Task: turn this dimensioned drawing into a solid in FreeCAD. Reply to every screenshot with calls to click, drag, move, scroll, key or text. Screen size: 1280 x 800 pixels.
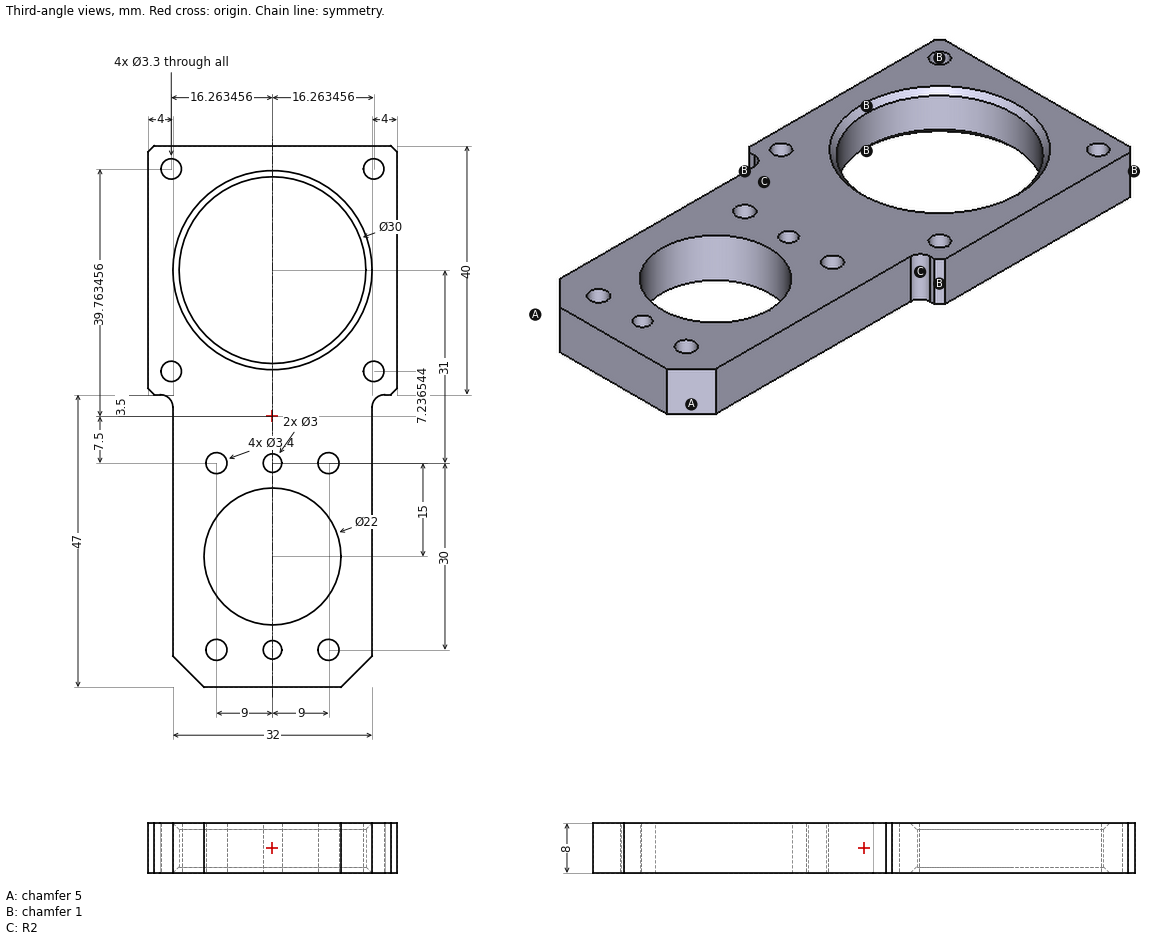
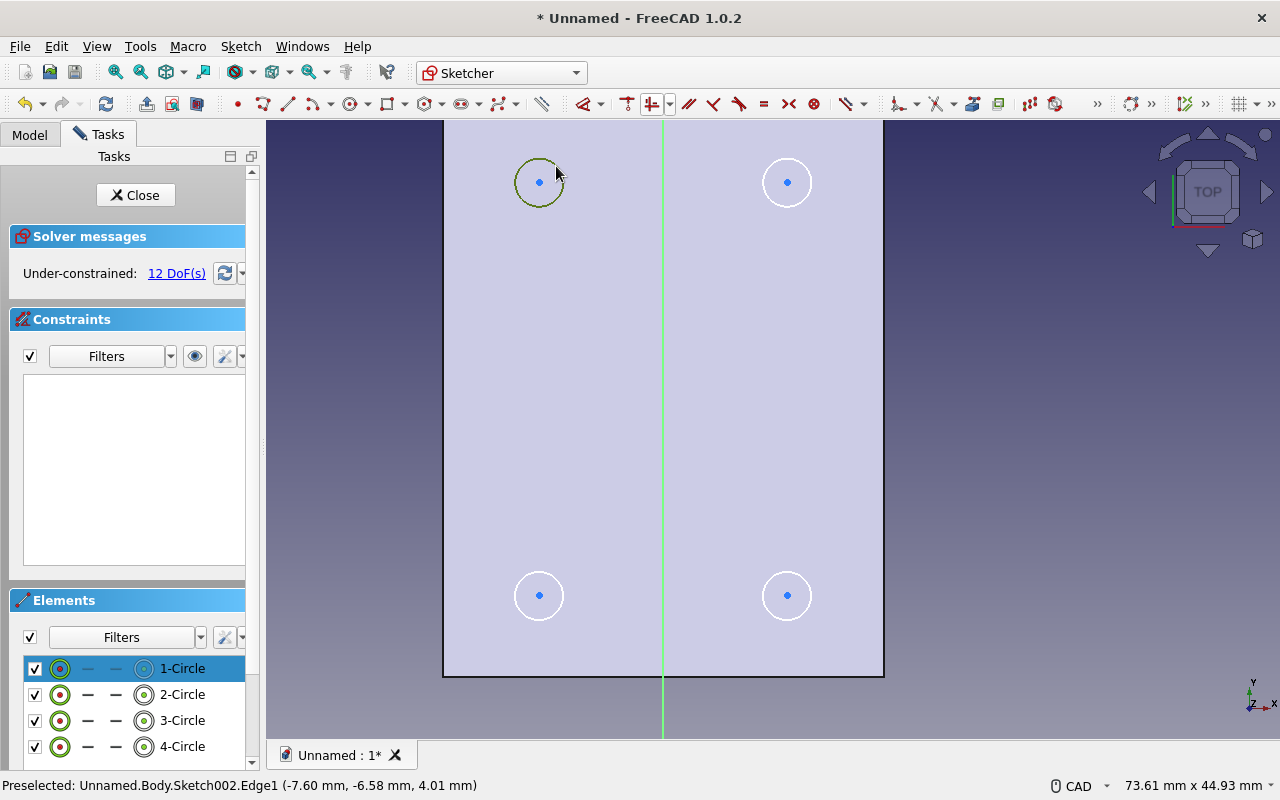
click(804, 166)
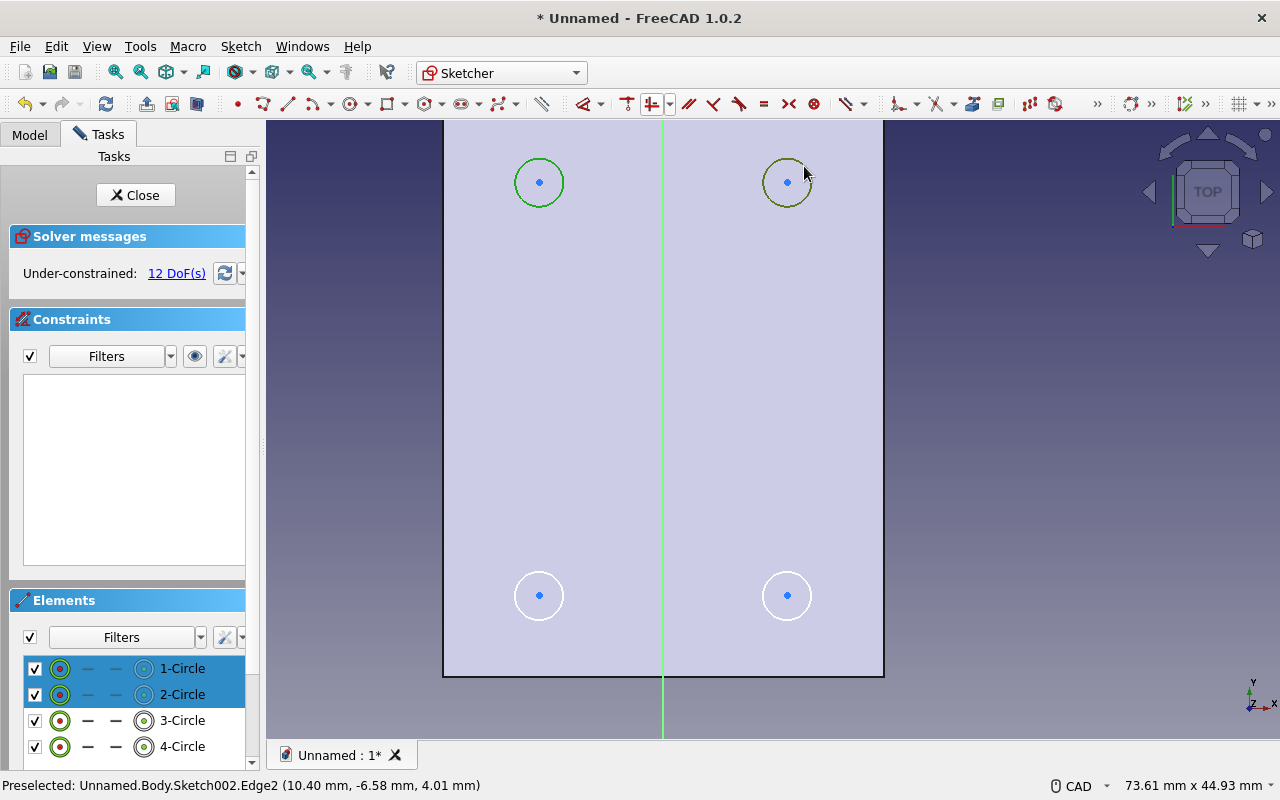
click(804, 579)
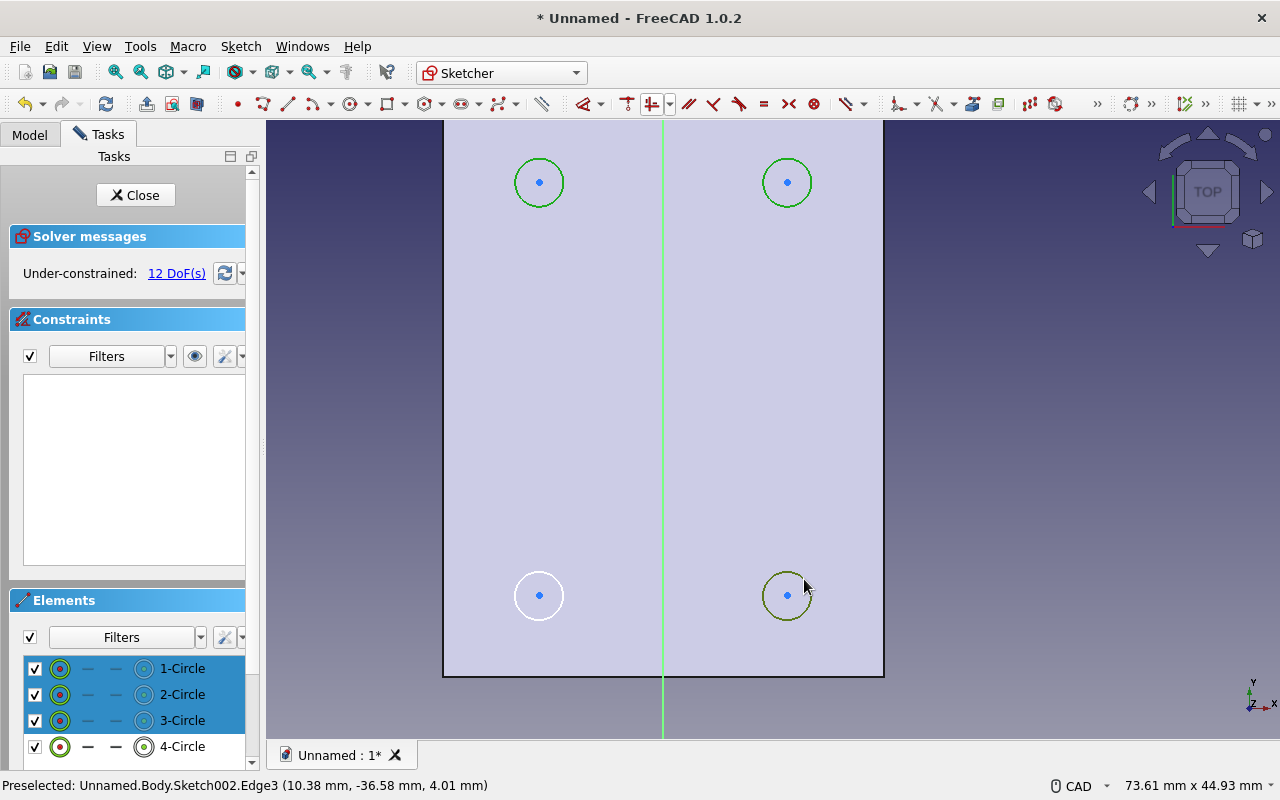
click(556, 579)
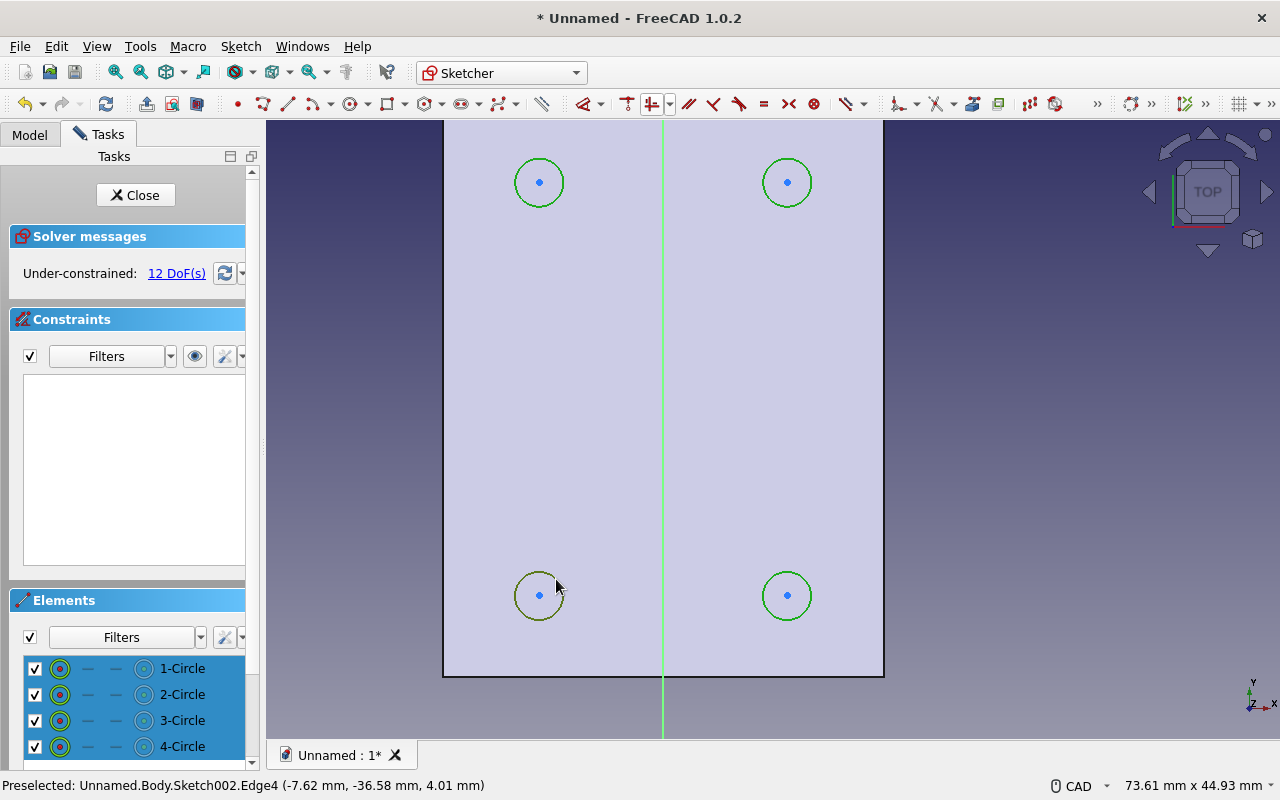
click(764, 104)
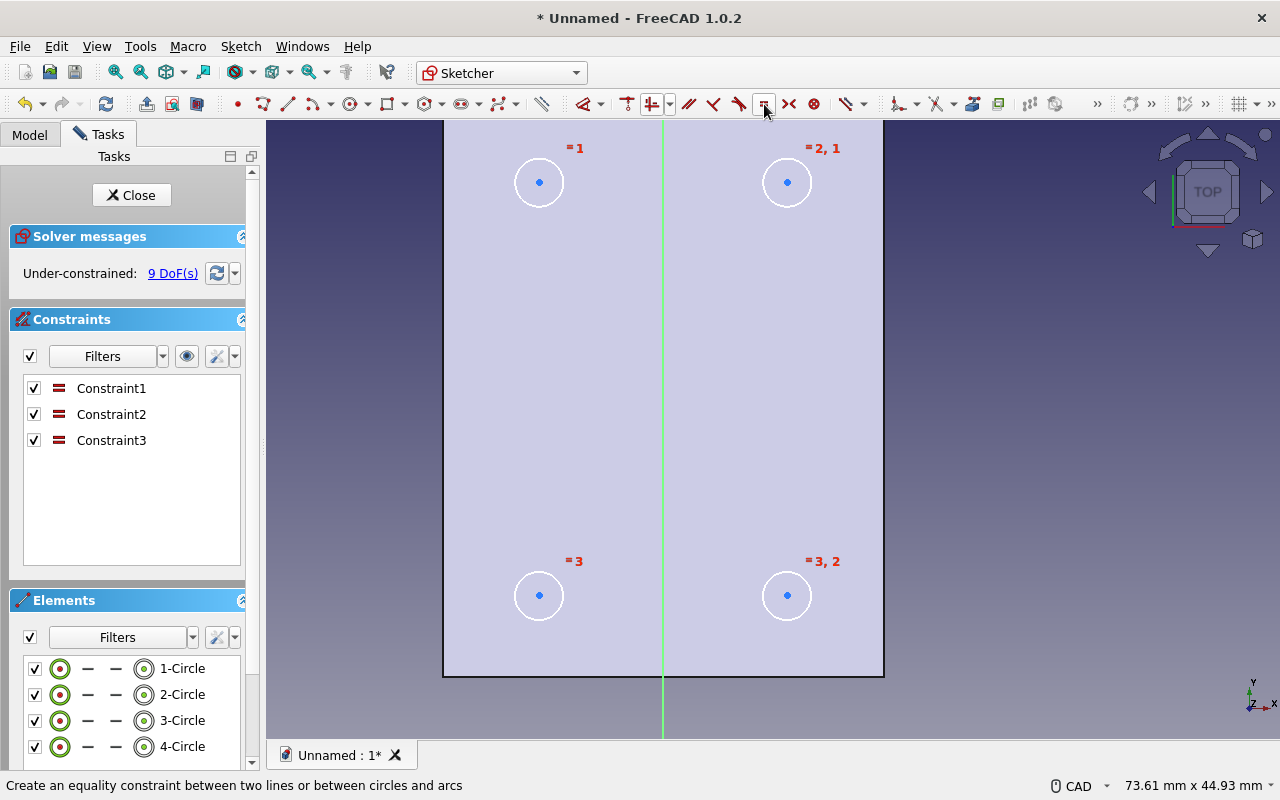
click(539, 183)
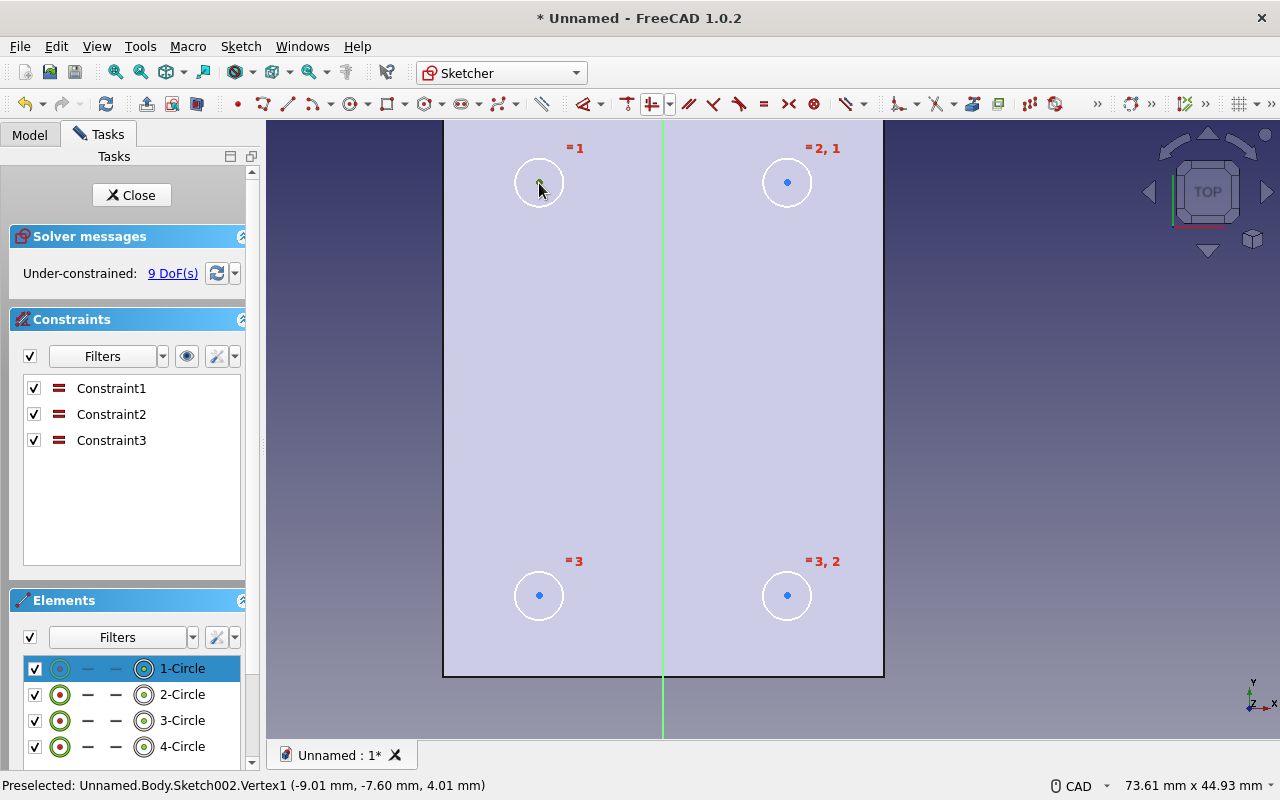
click(787, 183)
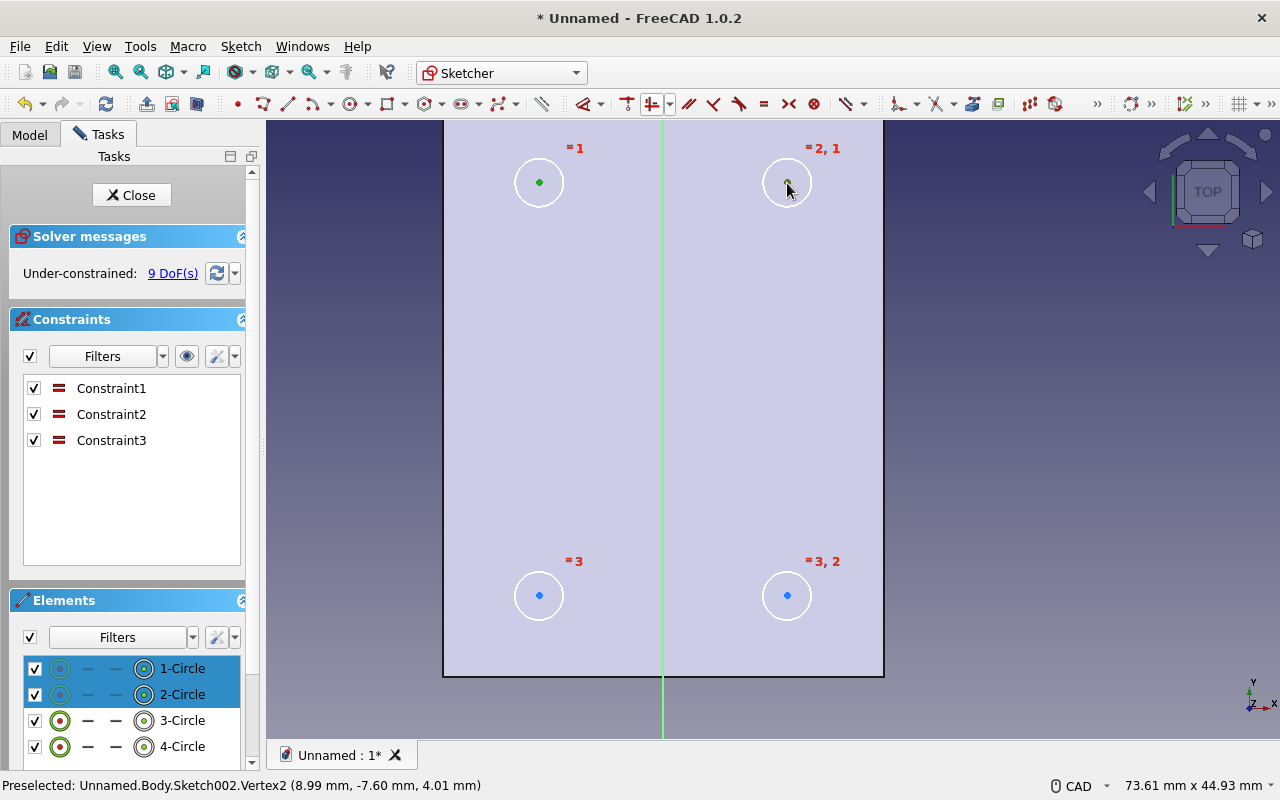
click(670, 104)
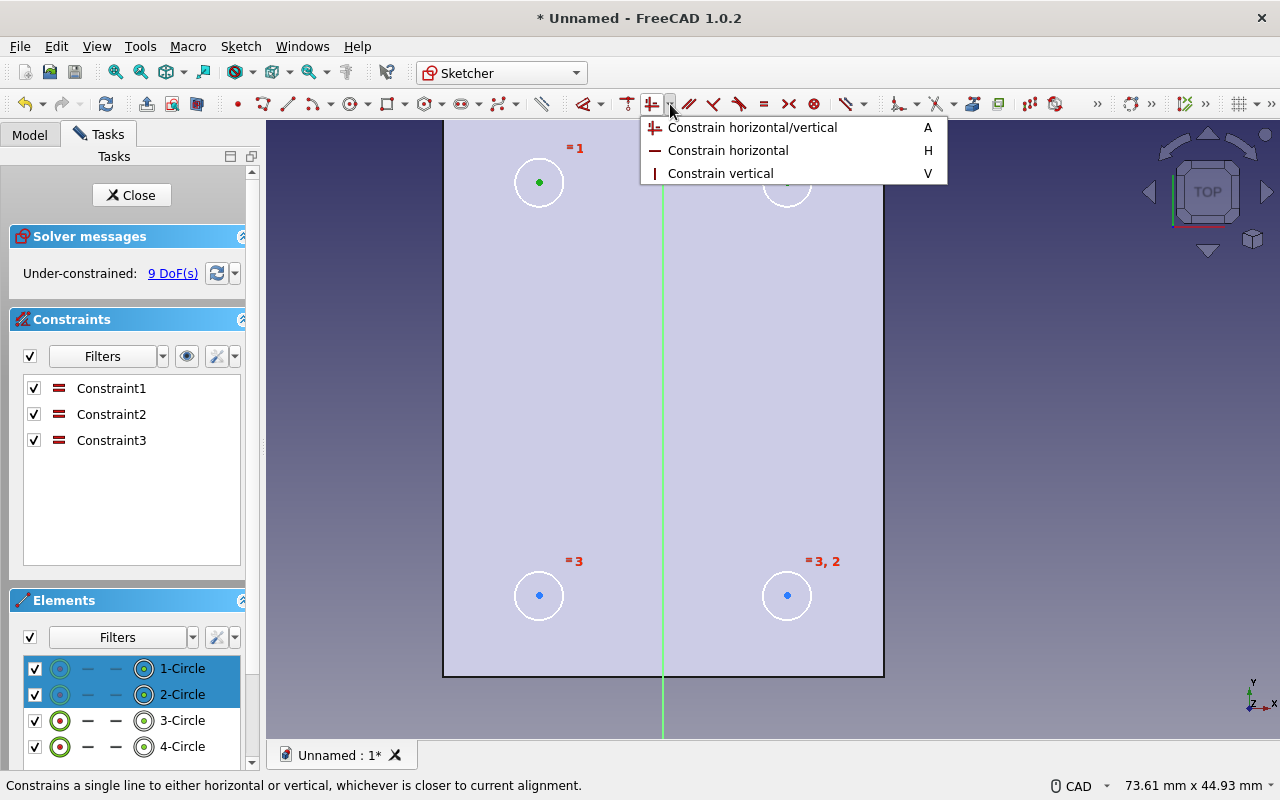
click(794, 150)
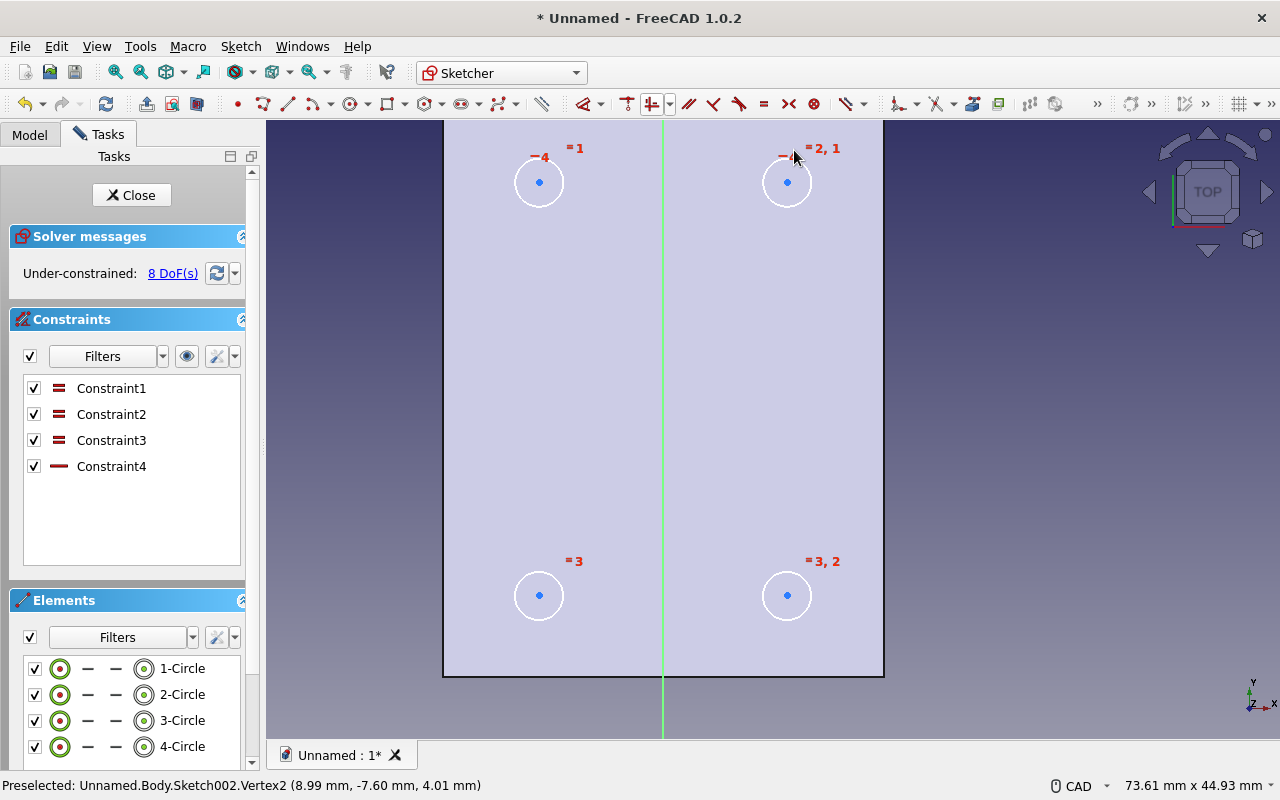
click(787, 183)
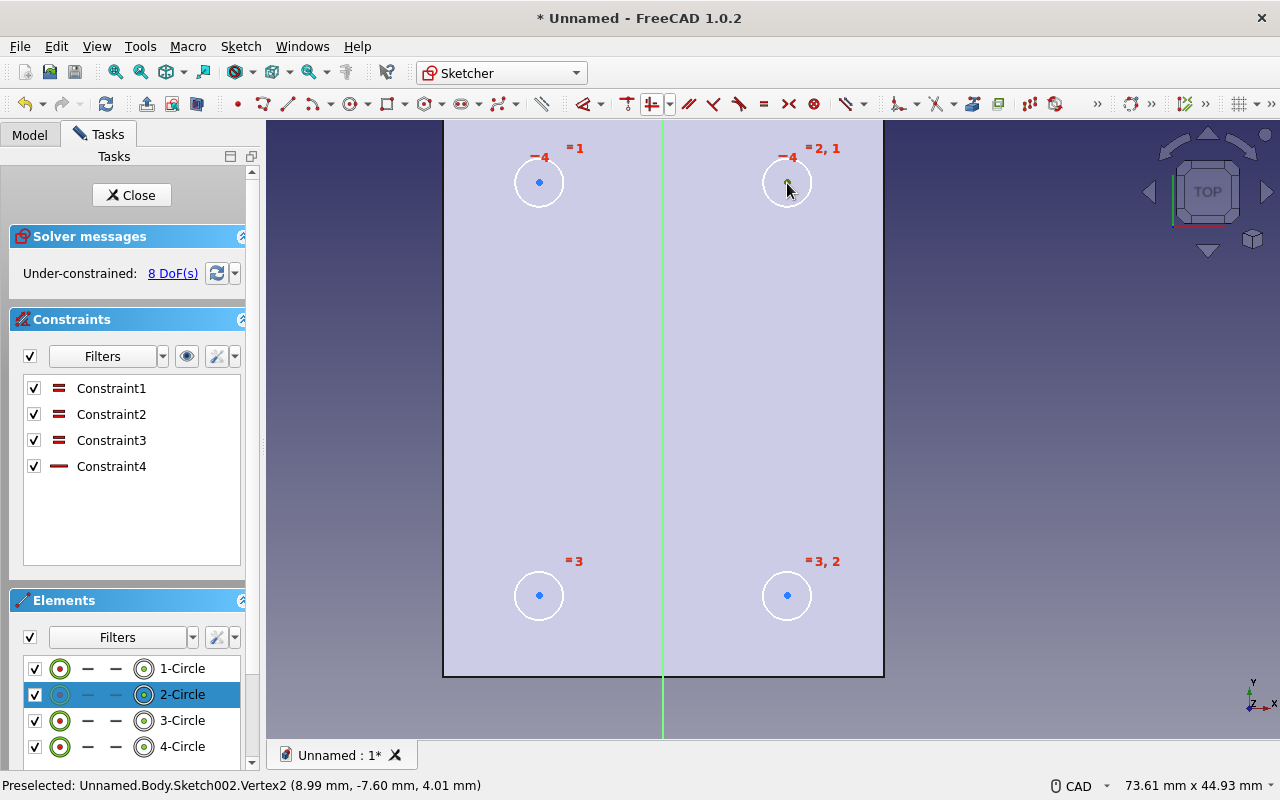
click(787, 596)